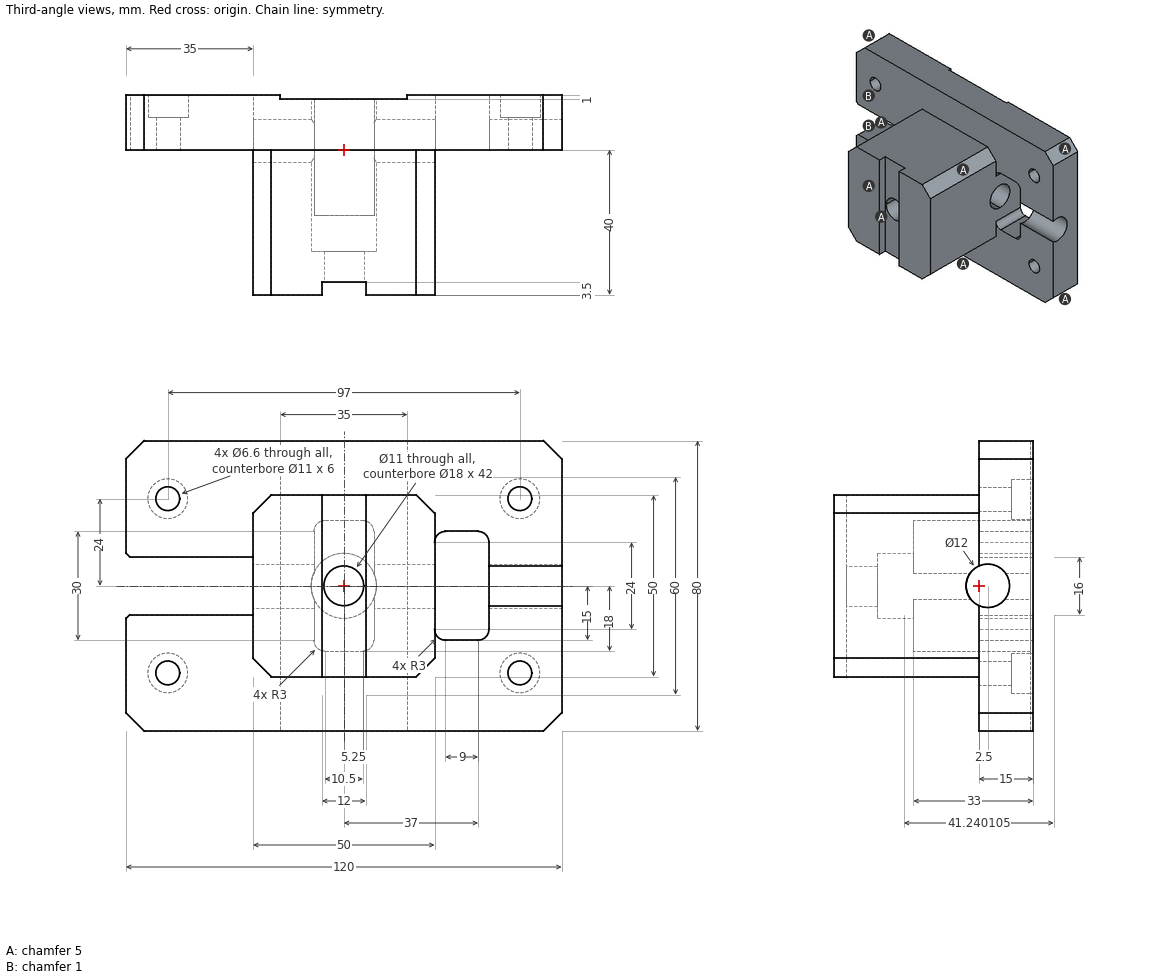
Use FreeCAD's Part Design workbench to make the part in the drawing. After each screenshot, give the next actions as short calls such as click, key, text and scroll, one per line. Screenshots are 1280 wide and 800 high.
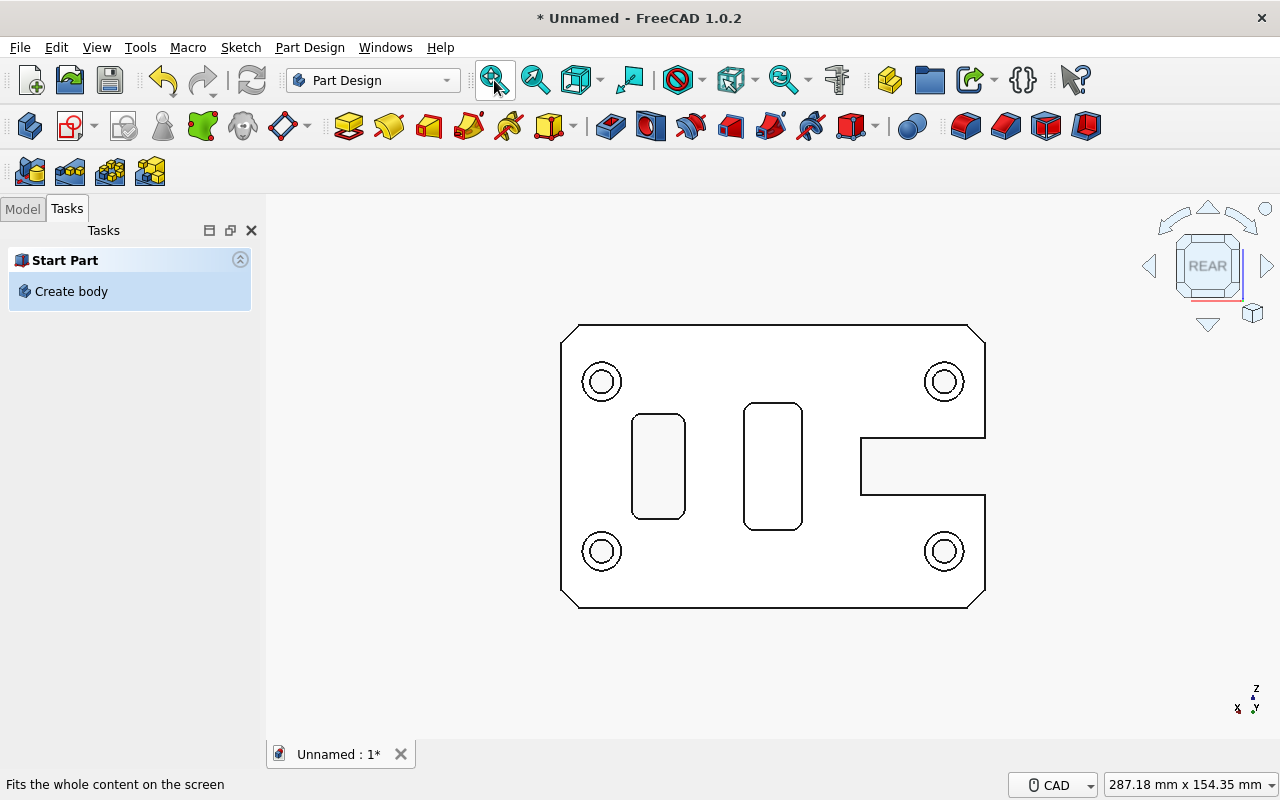
key(6)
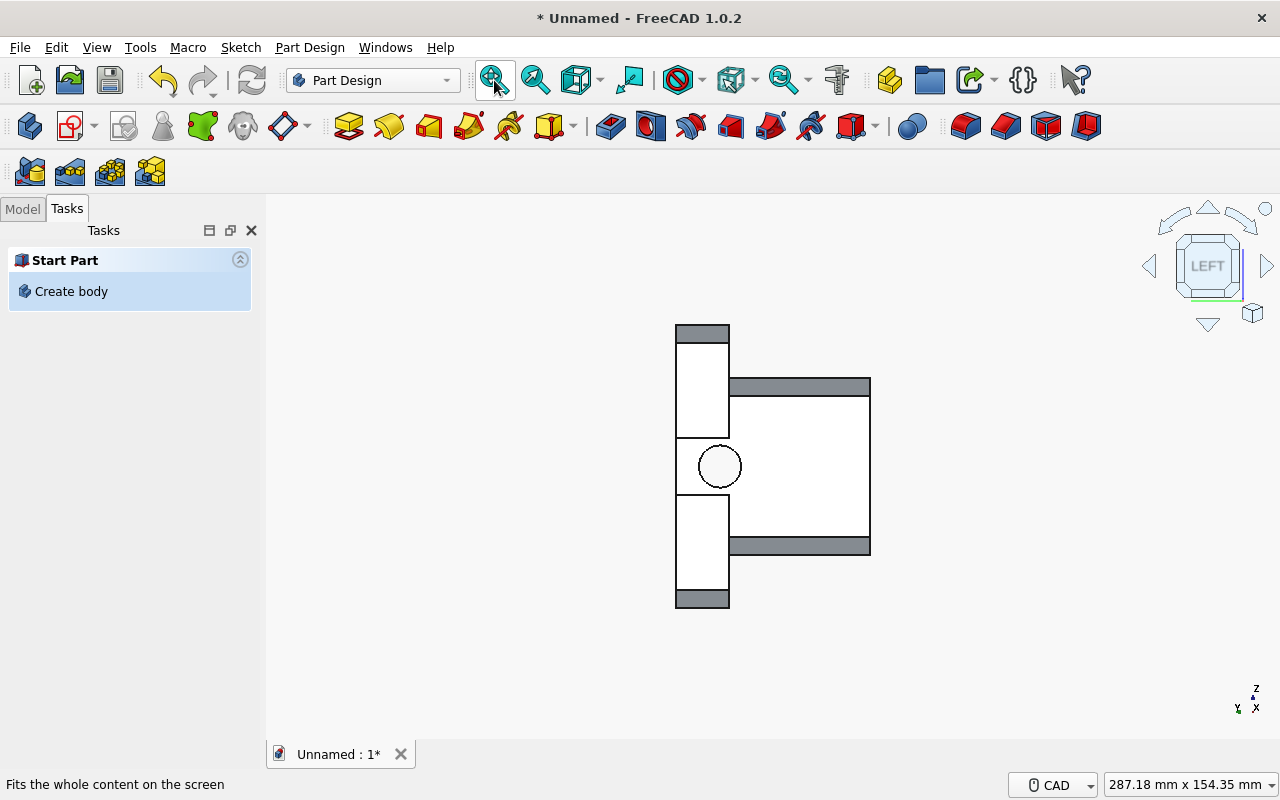
click(702, 494)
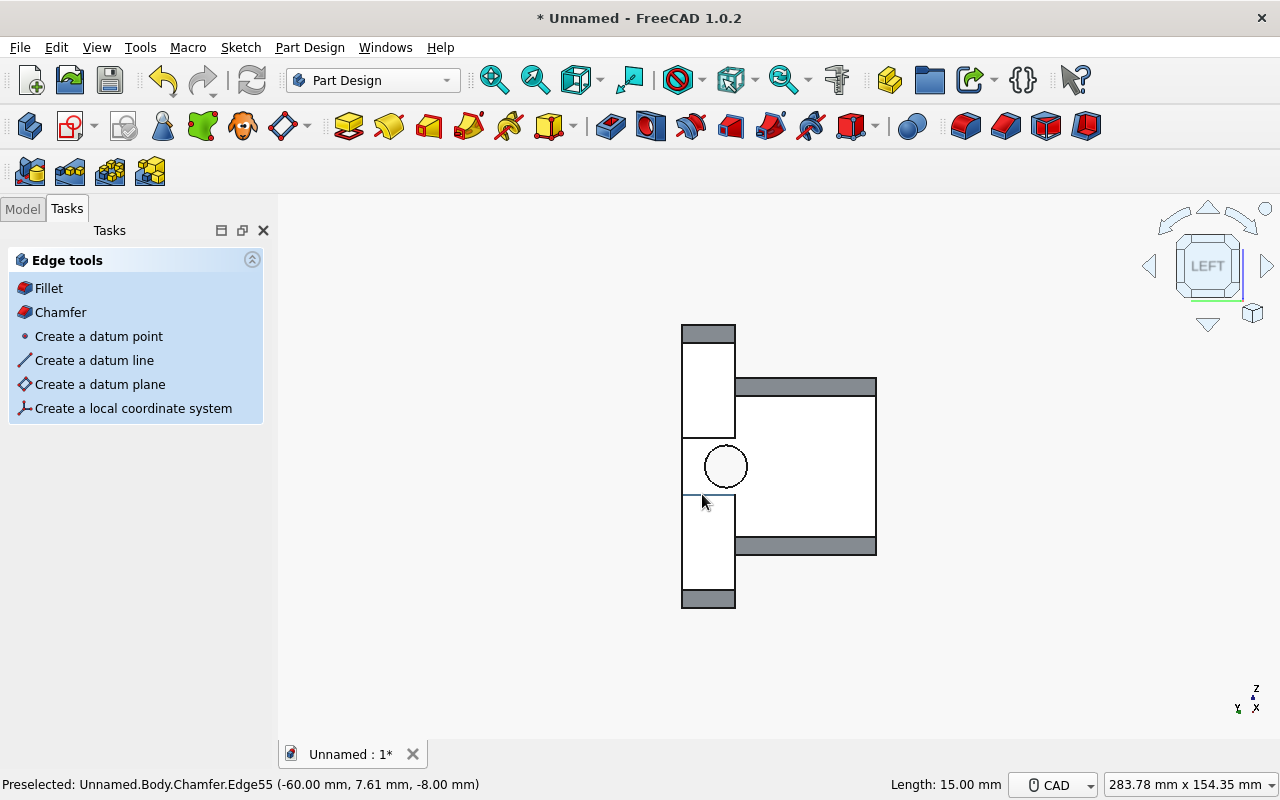
click(708, 437, ctrl)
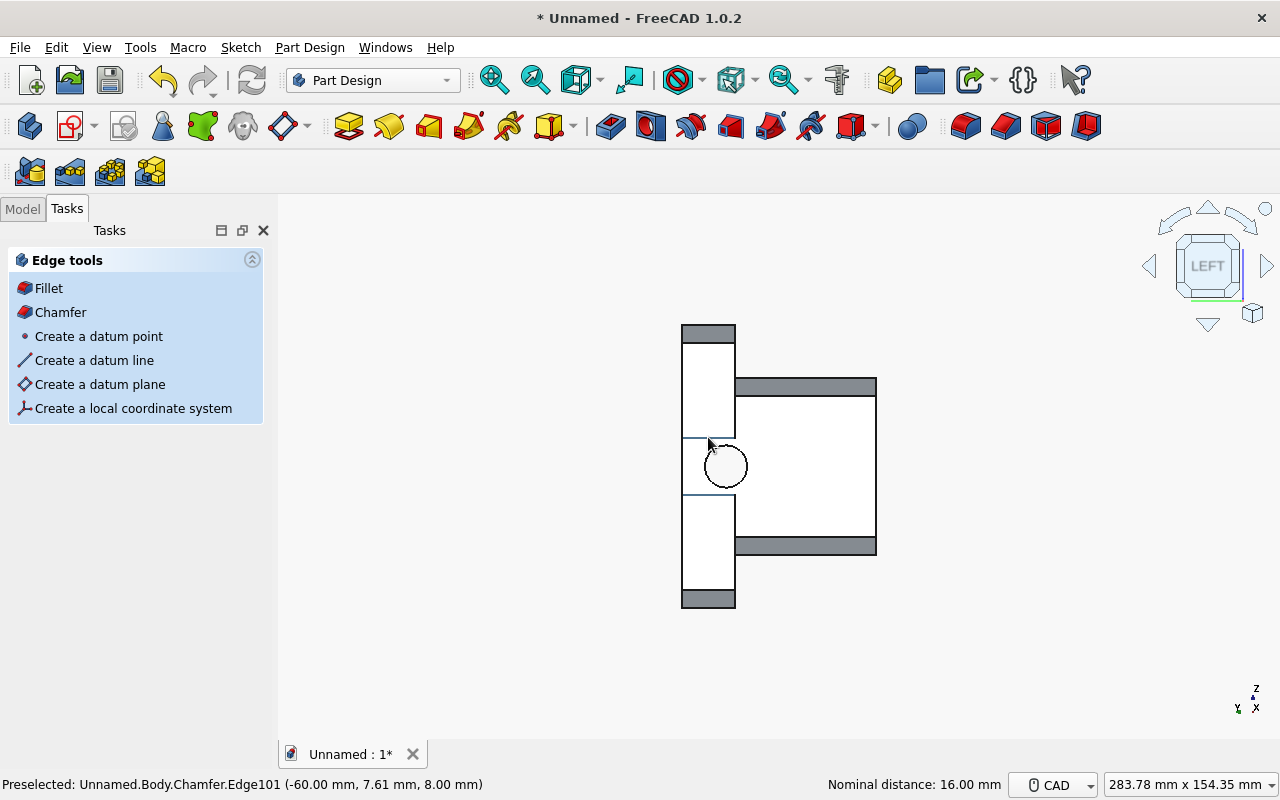
click(1006, 126)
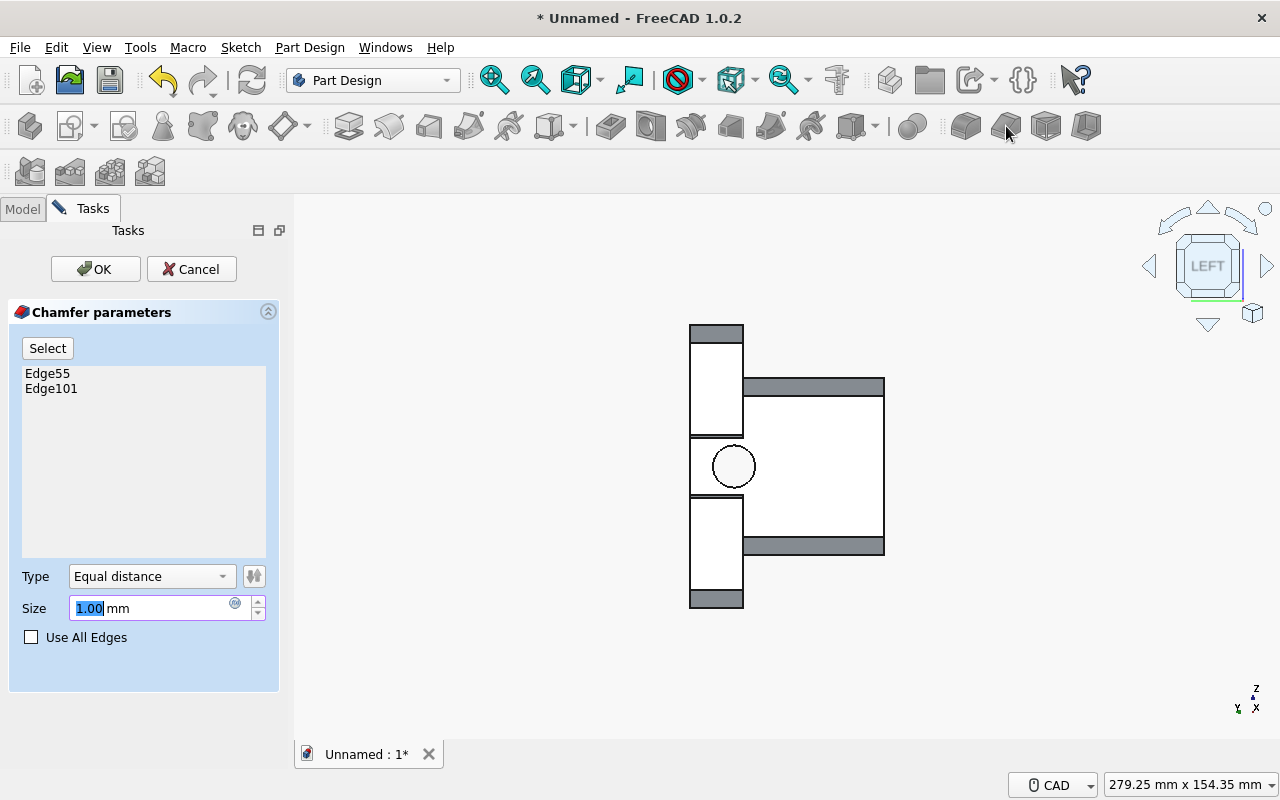
text(1)
key(Tab)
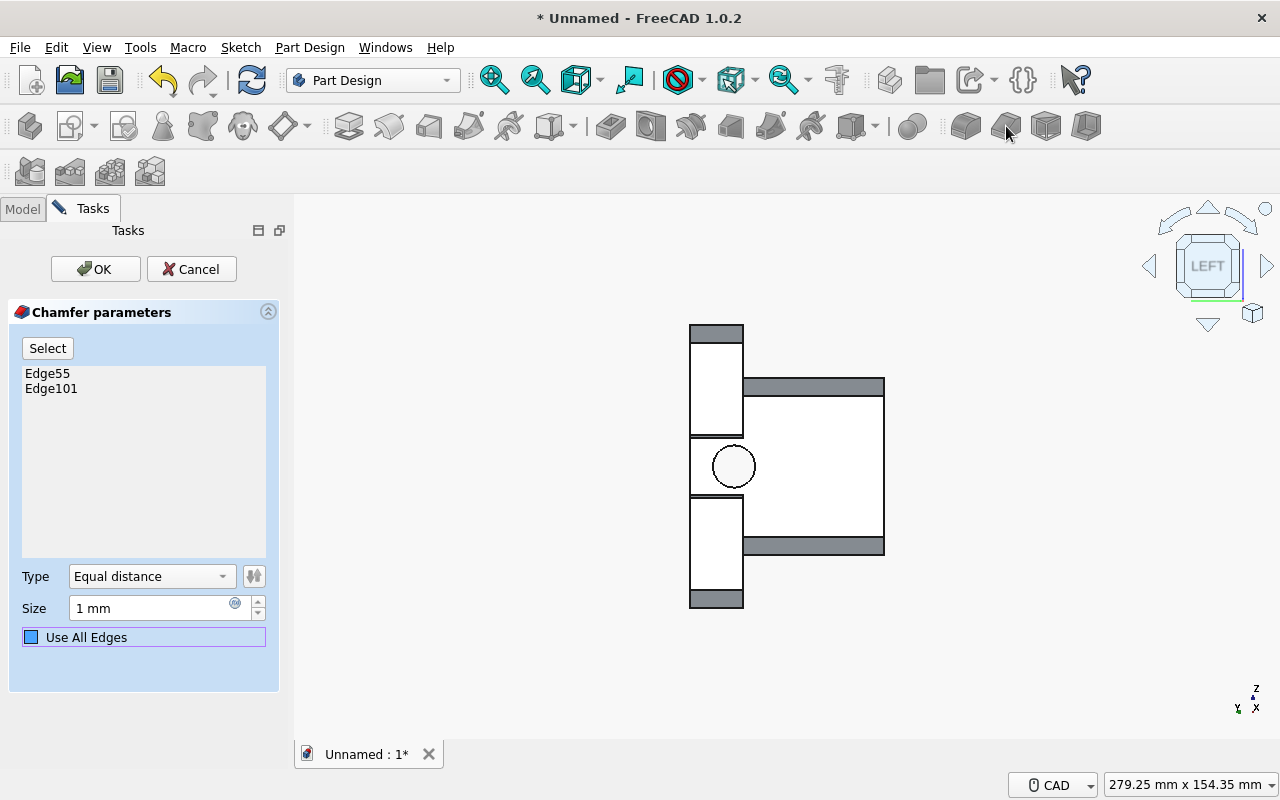
click(96, 269)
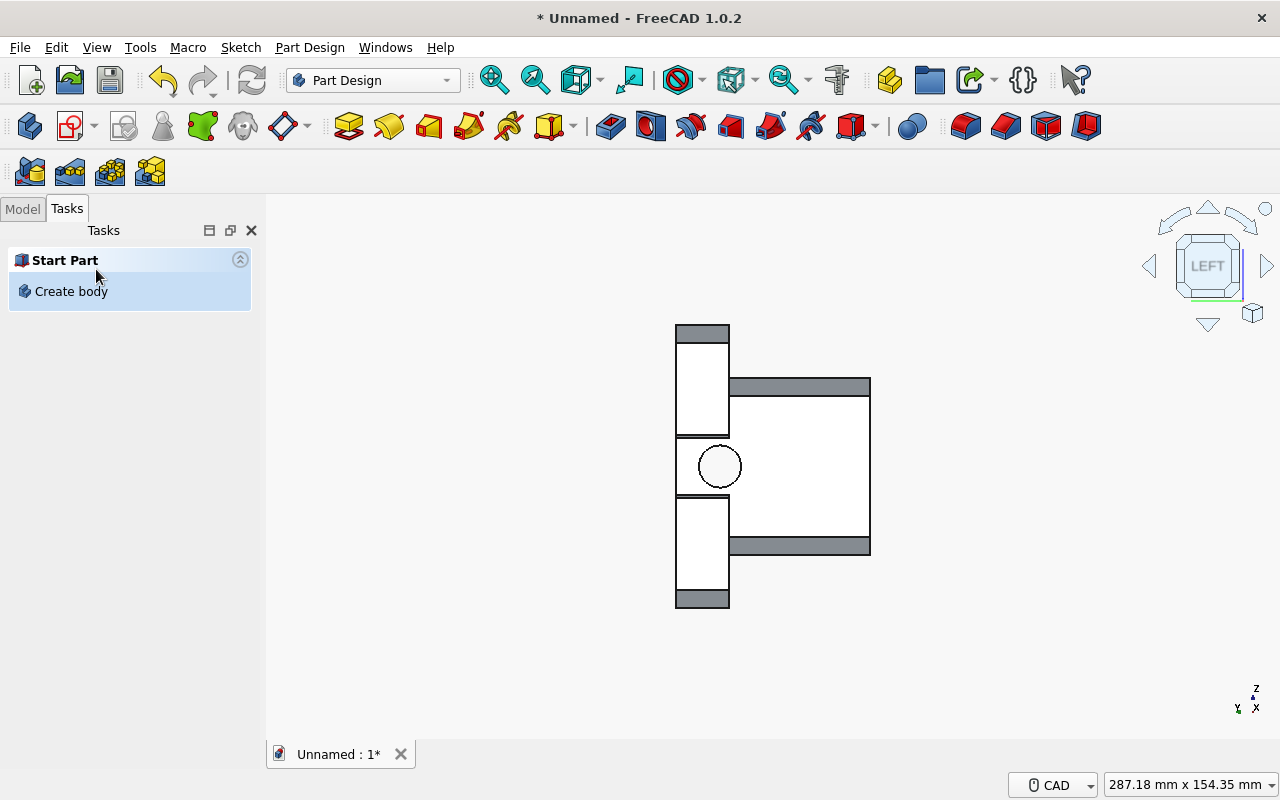
key(4)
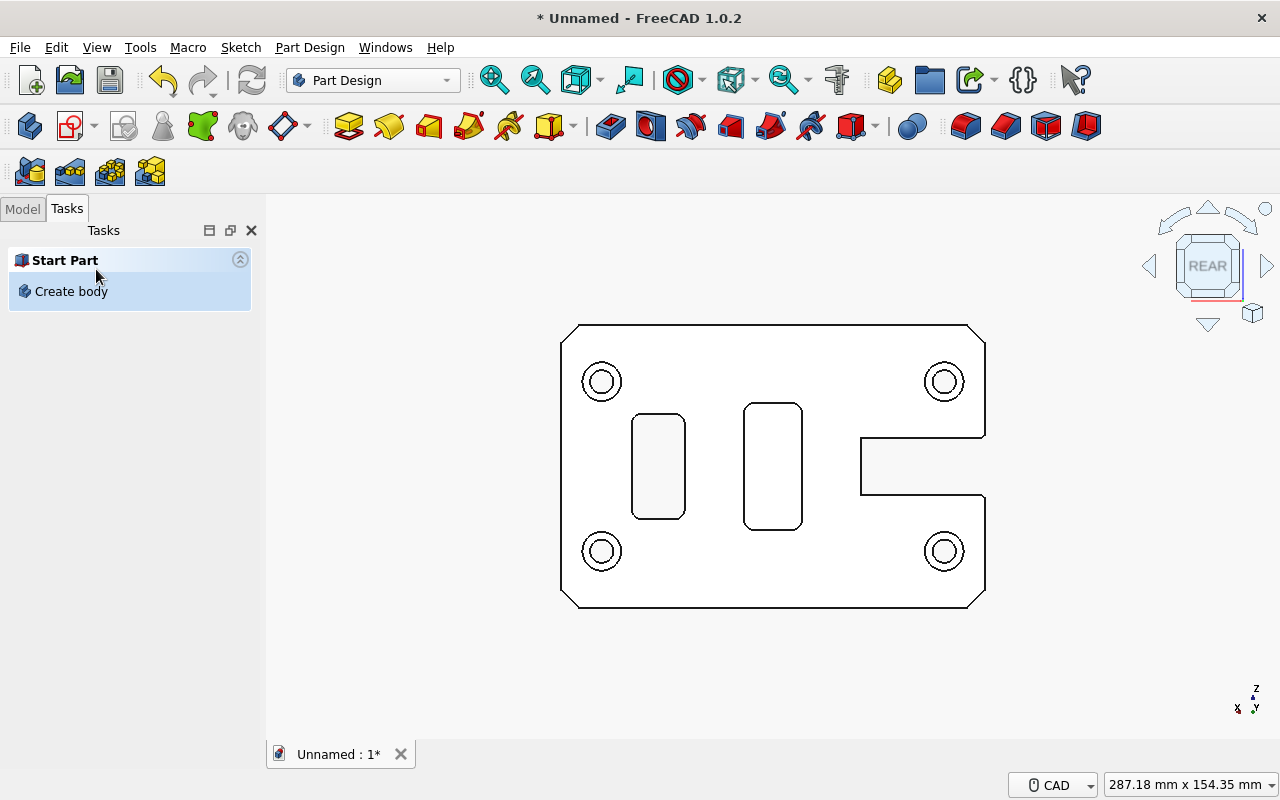
click(712, 546)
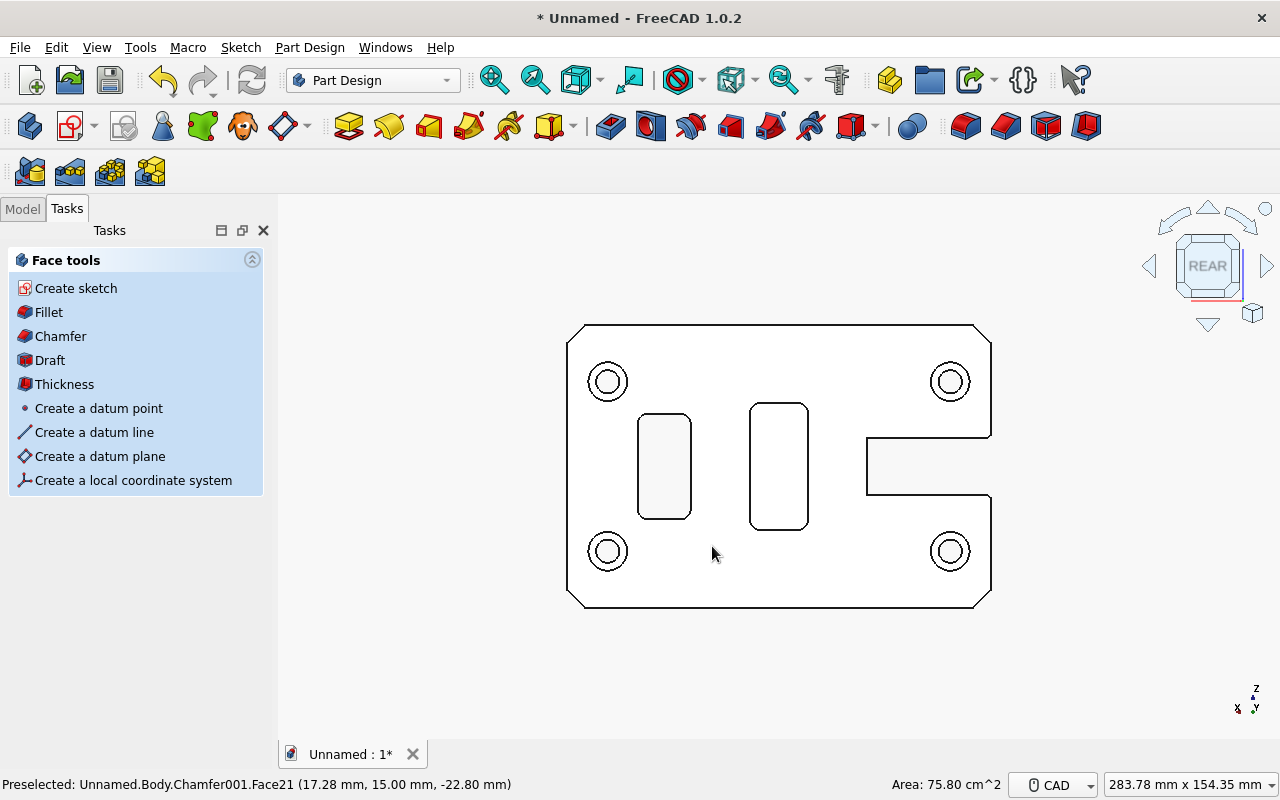
click(70, 126)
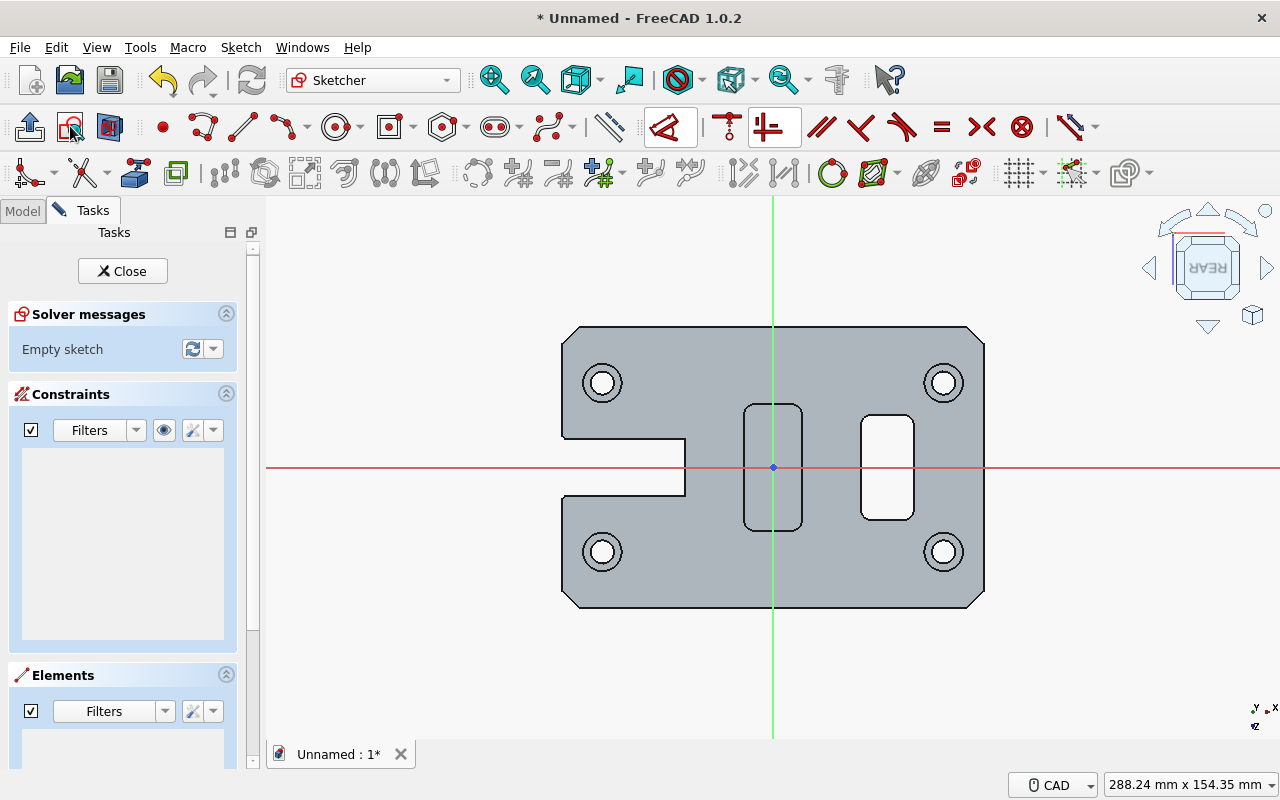
click(390, 128)